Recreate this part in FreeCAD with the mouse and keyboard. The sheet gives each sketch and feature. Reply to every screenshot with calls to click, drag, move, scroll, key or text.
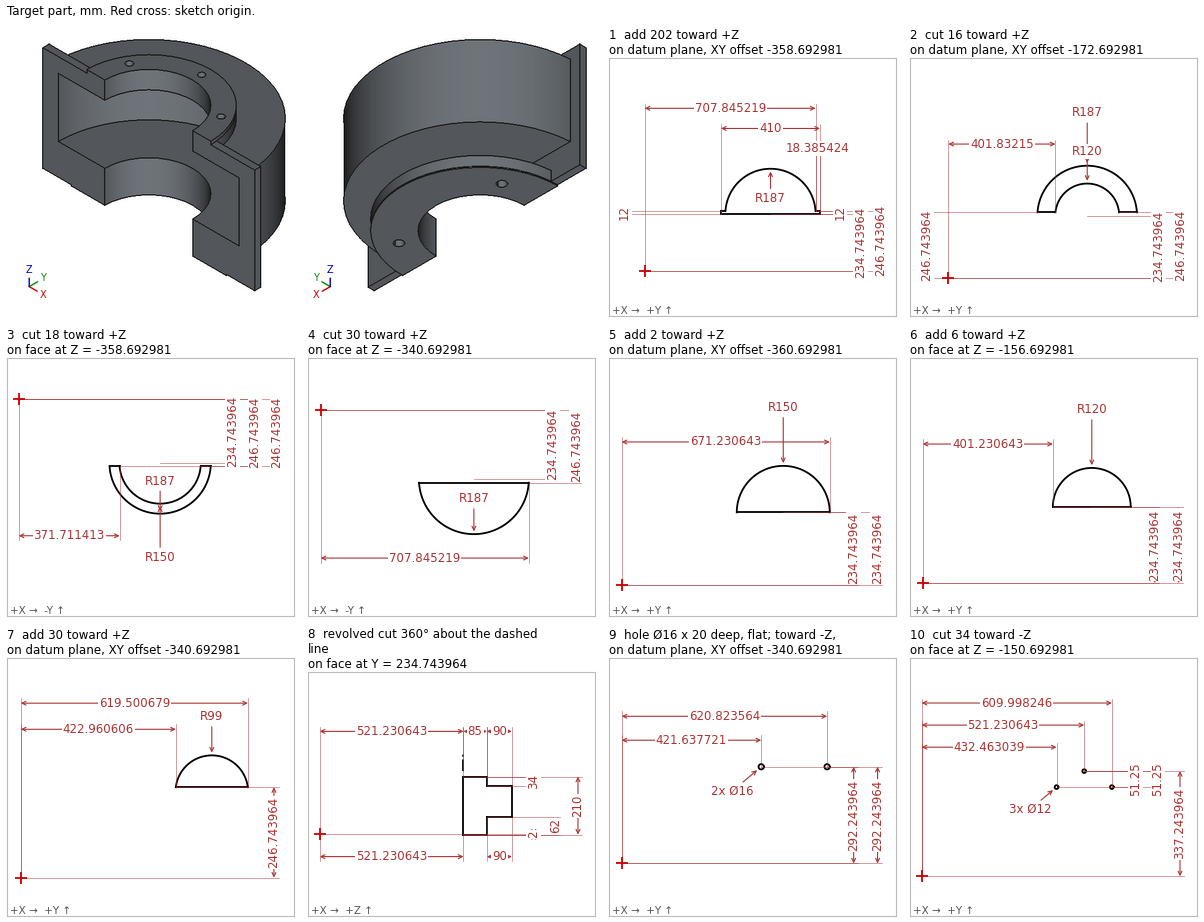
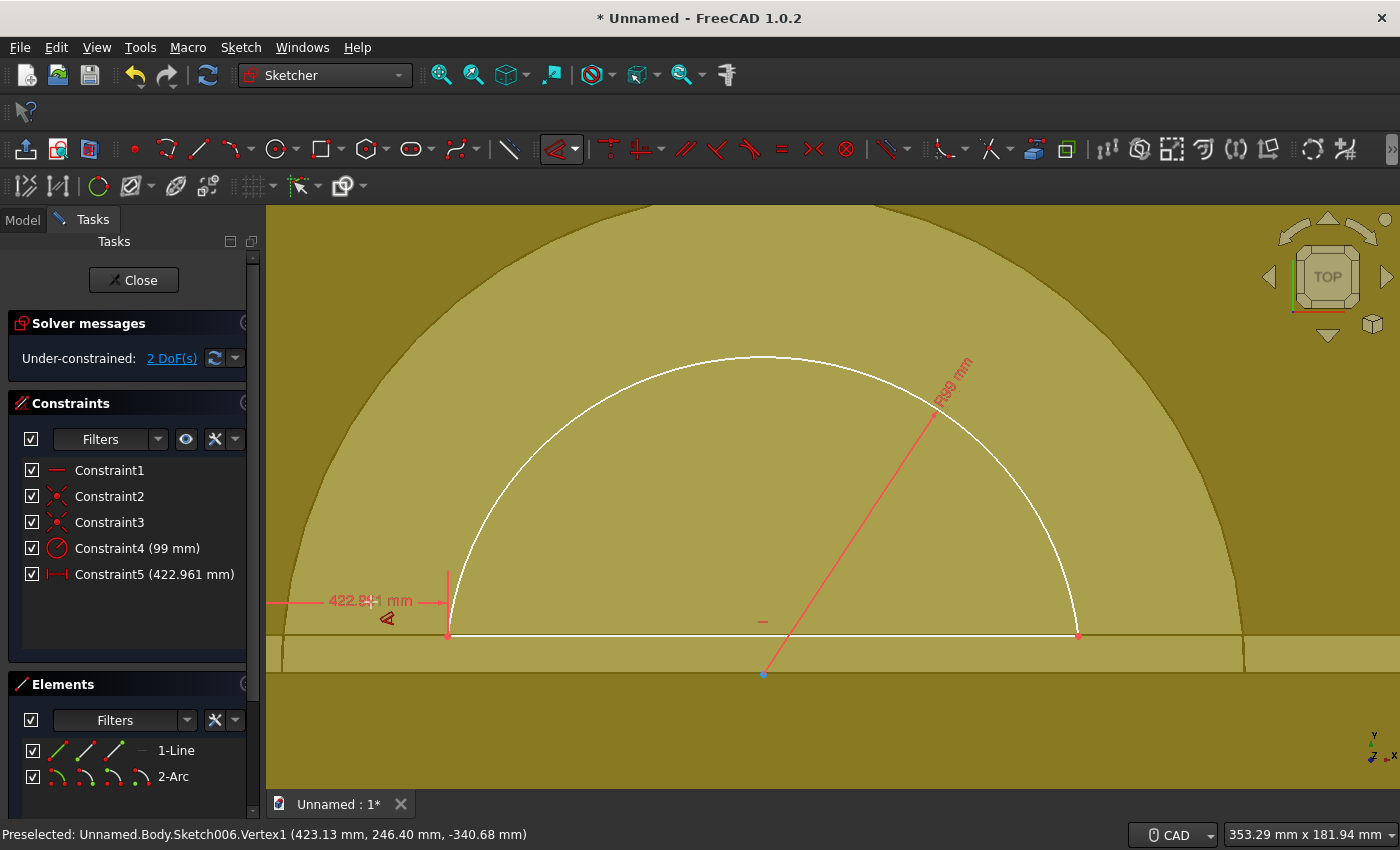
click(448, 636)
click(482, 699)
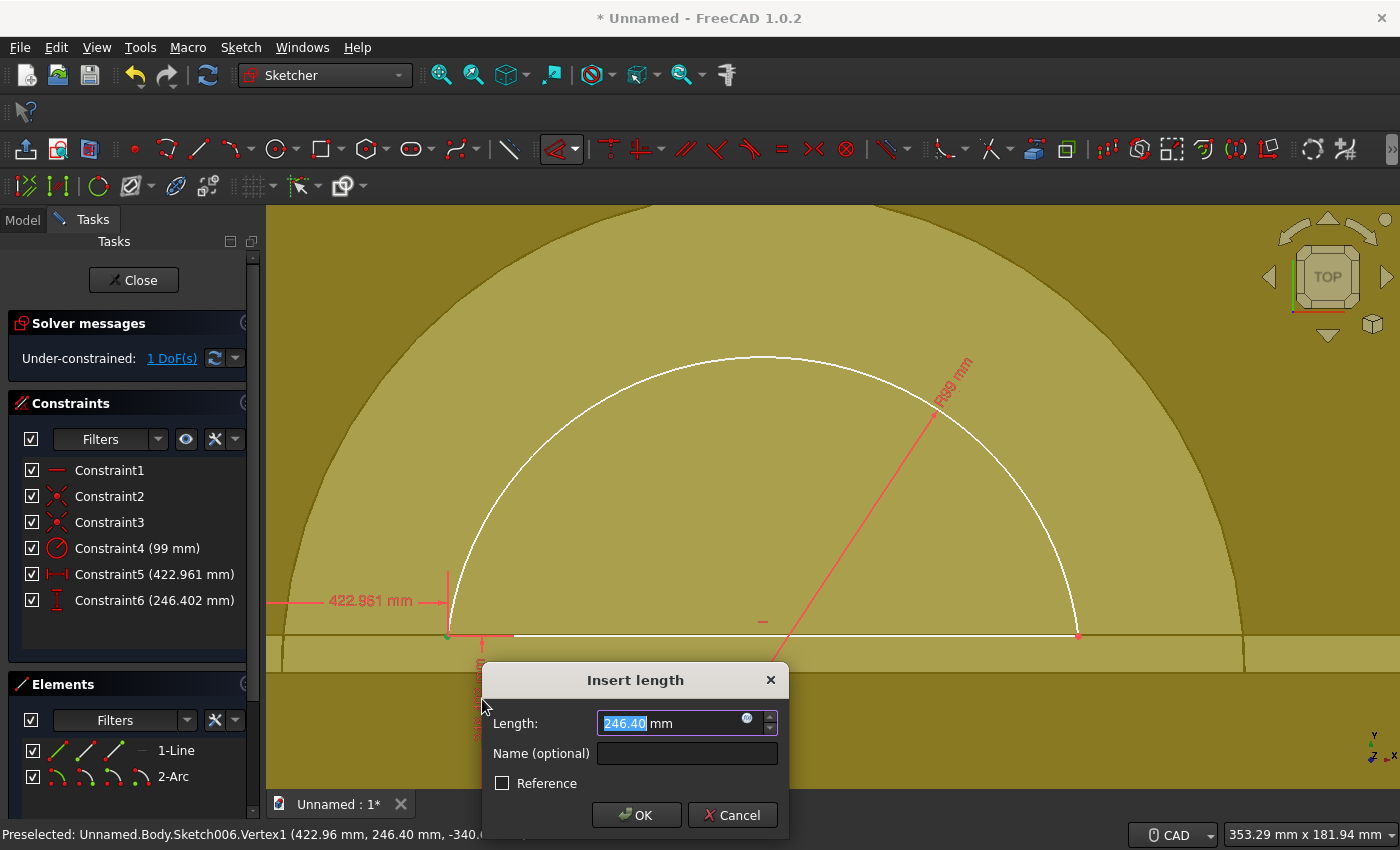
text(246.743964)
key(Return)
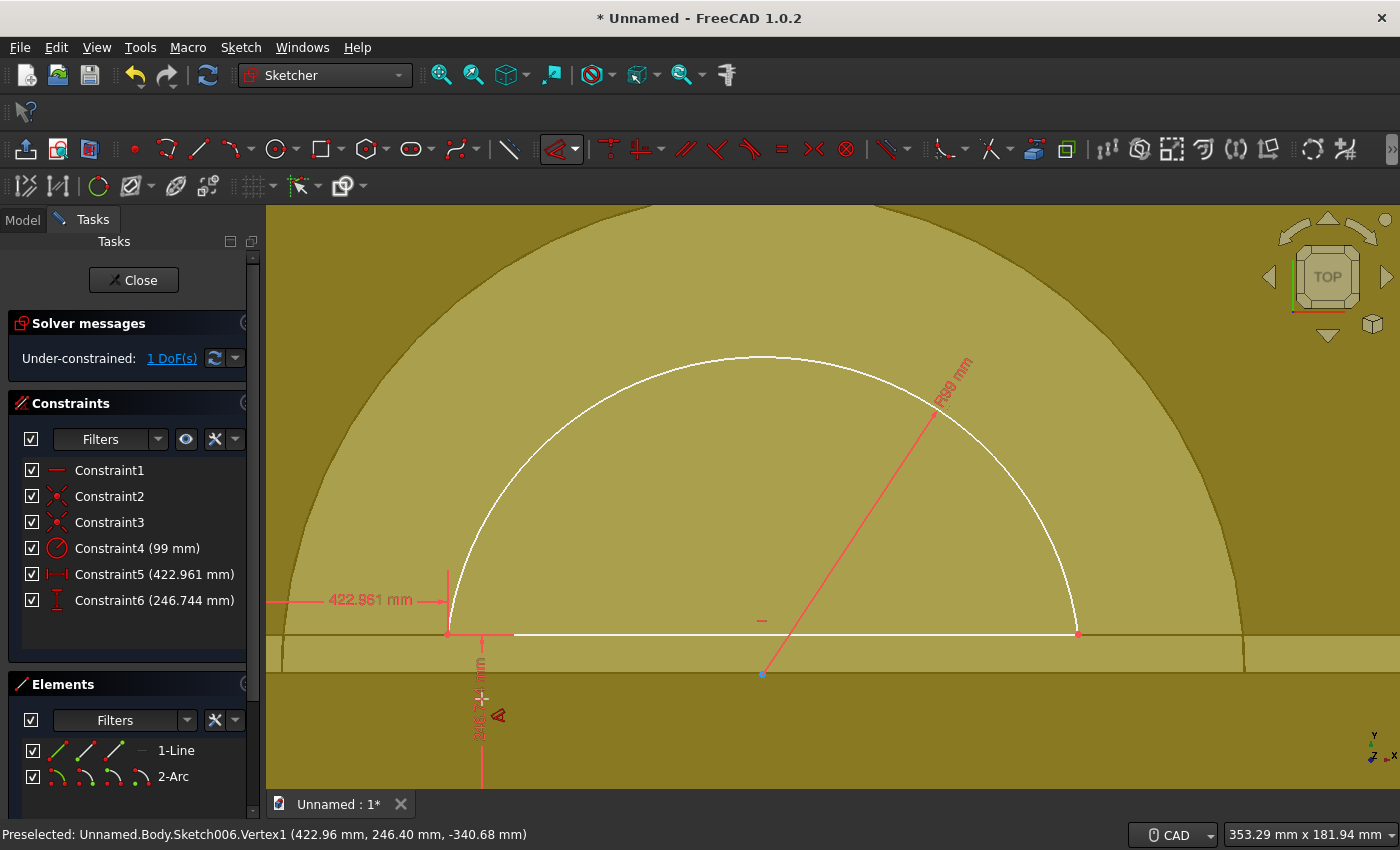
click(1078, 635)
click(686, 601)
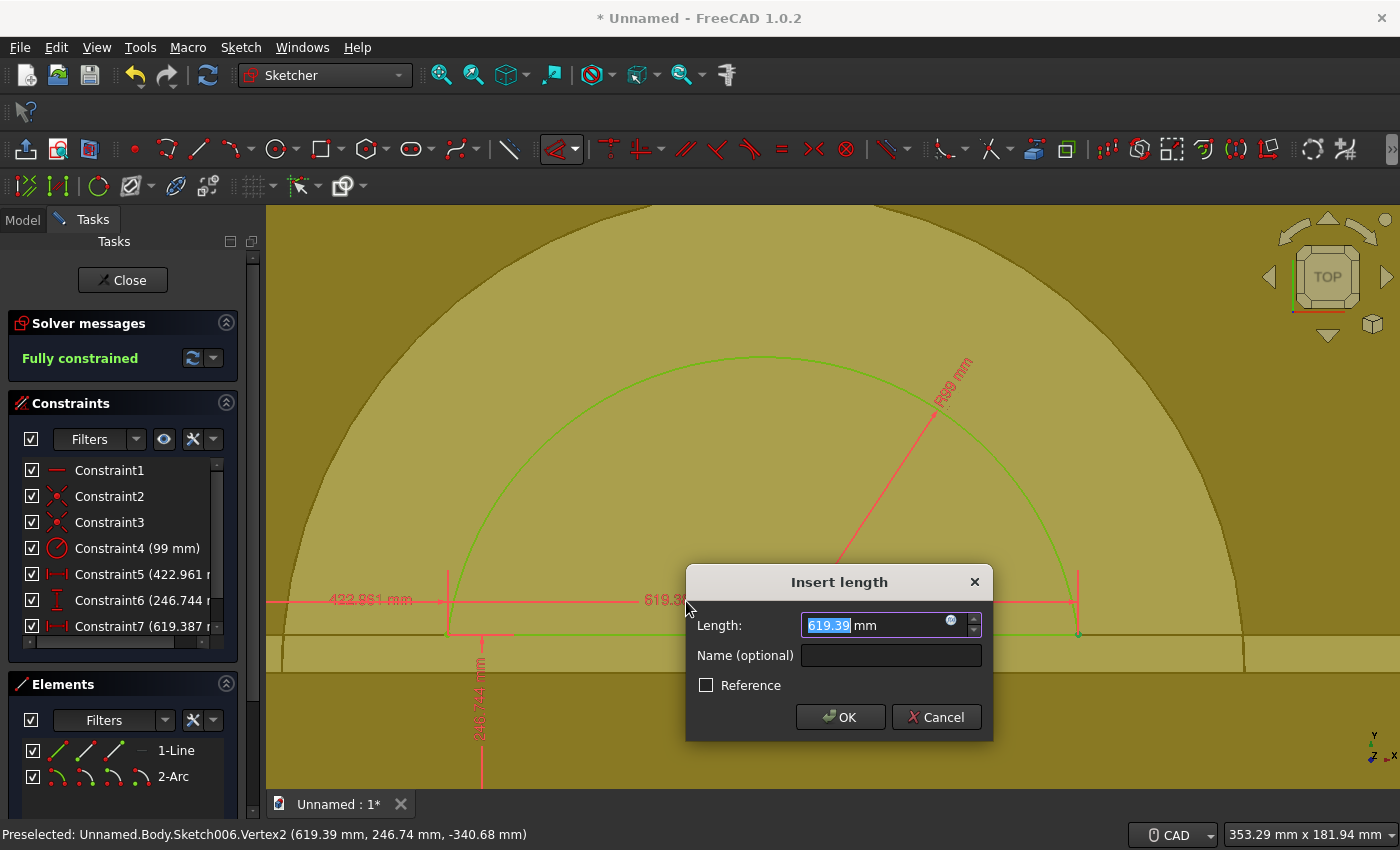
text(619.500679)
key(Return)
key(Escape)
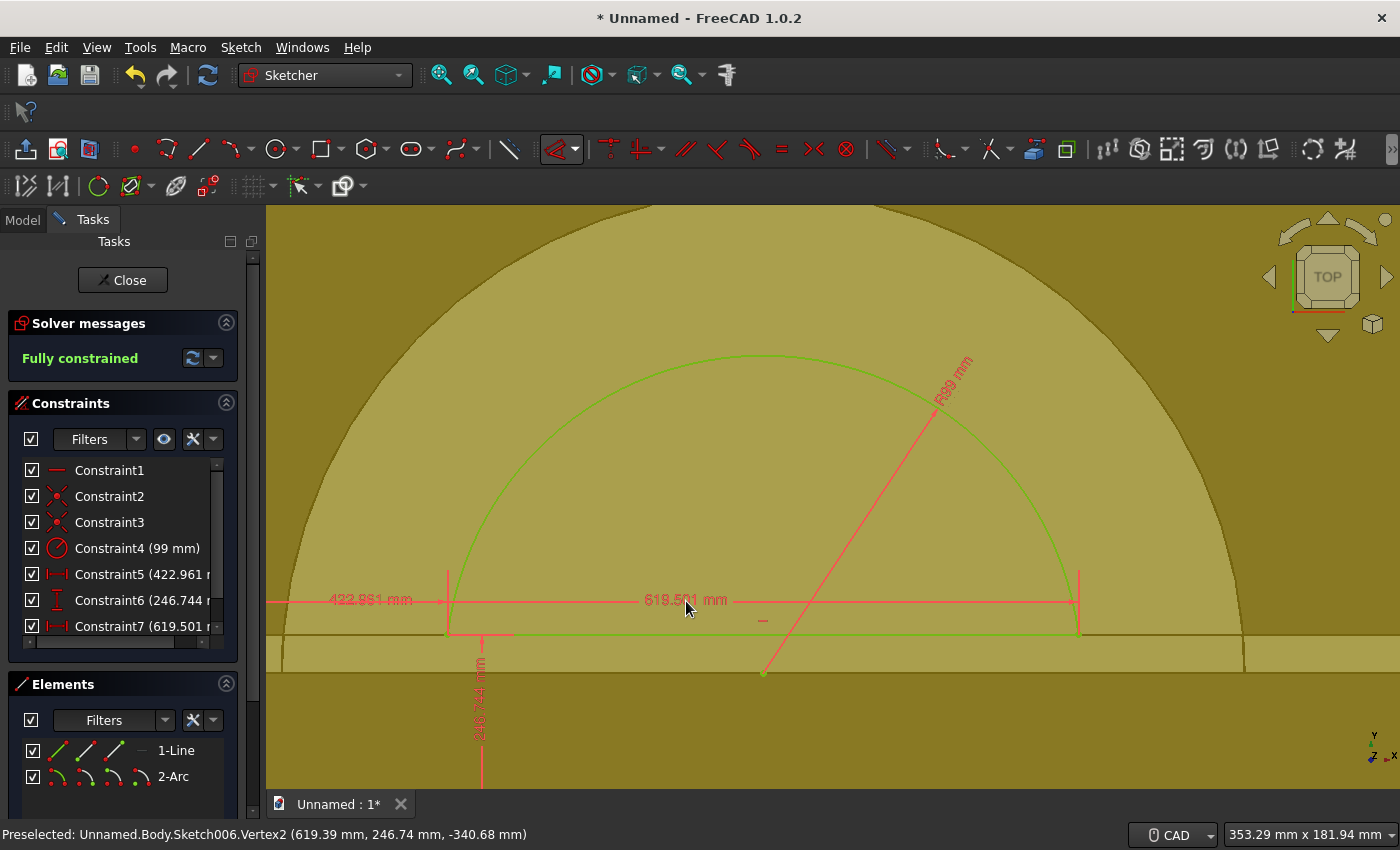
click(123, 280)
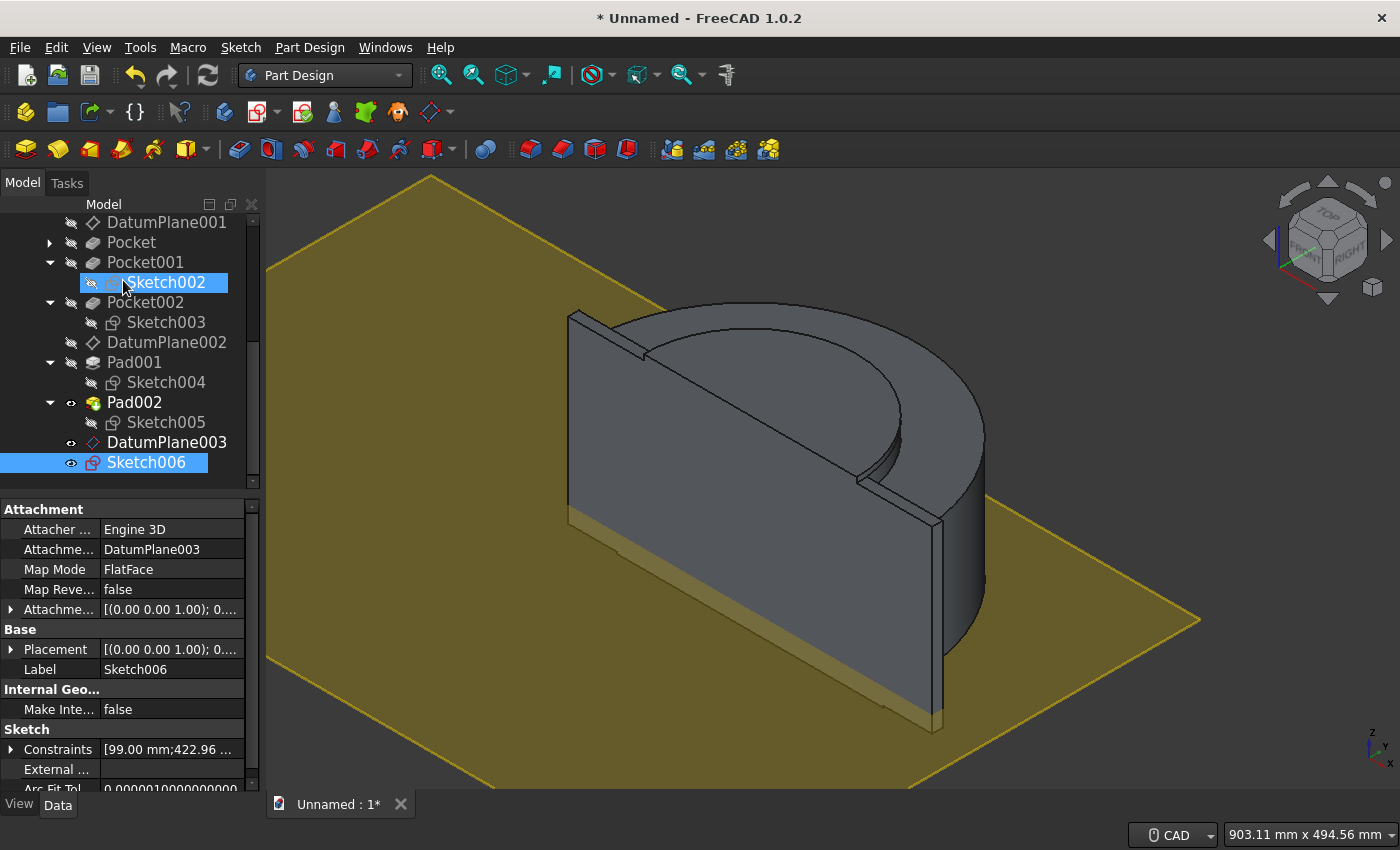
click(26, 150)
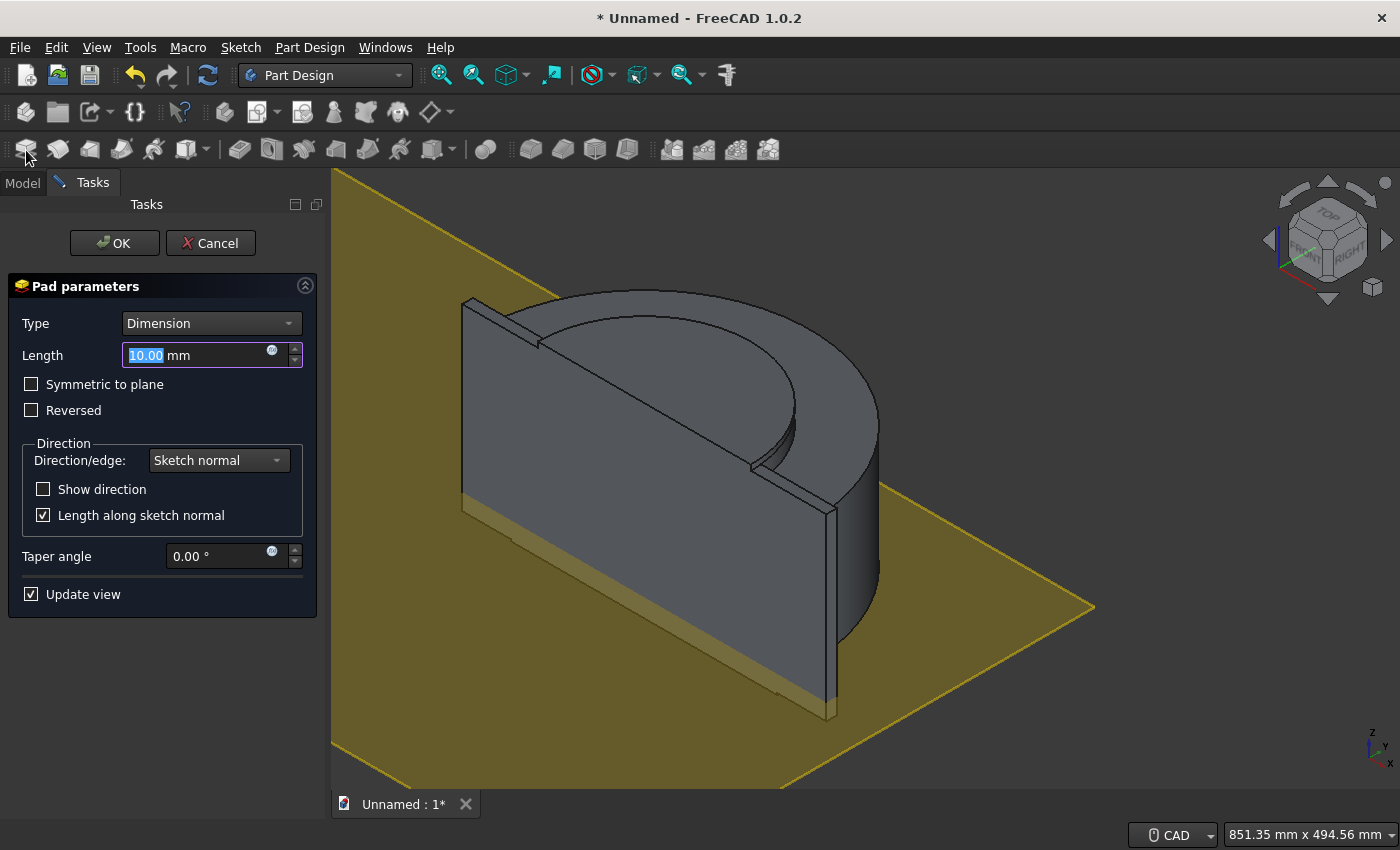
text(30)
key(Tab)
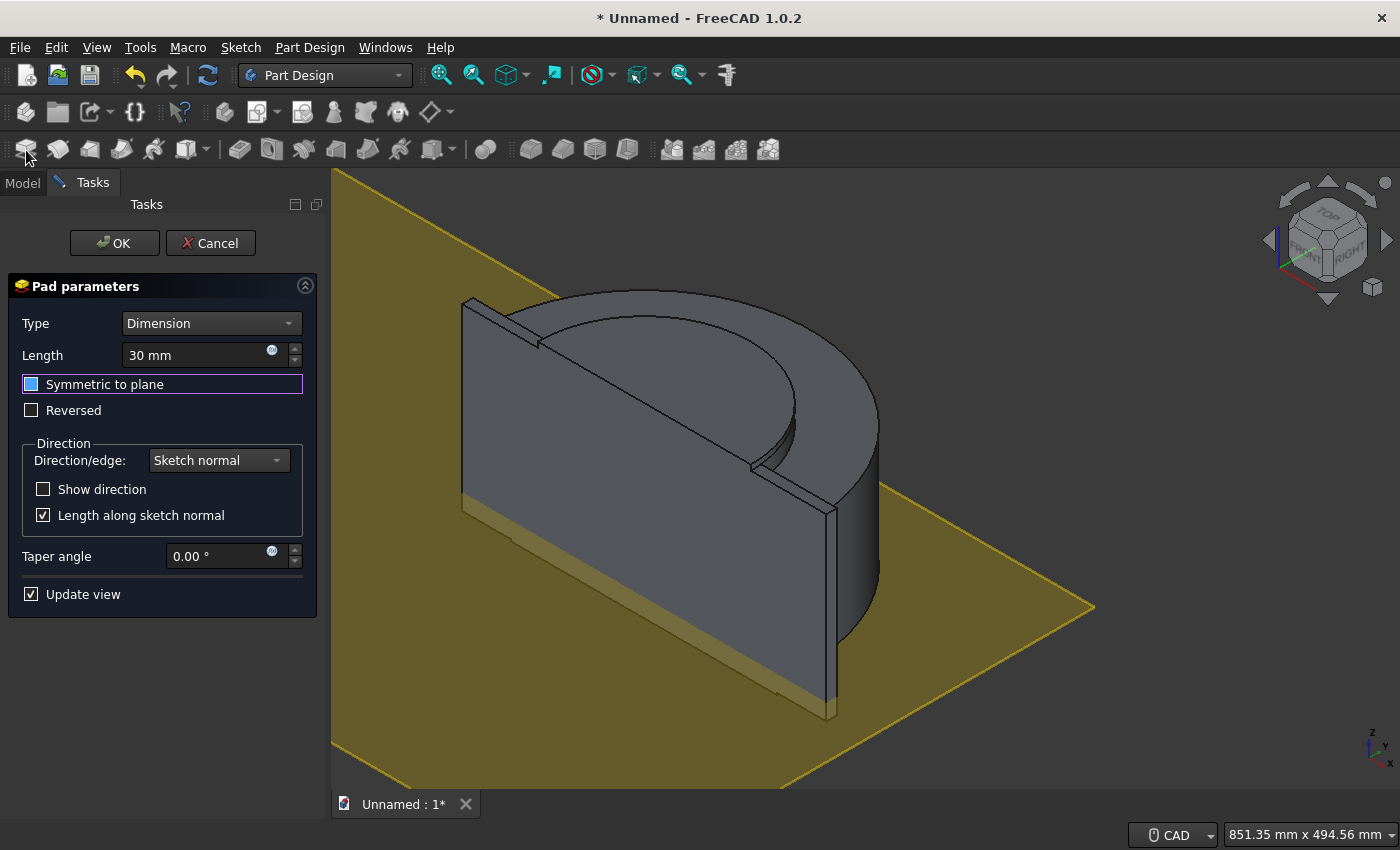
click(115, 243)